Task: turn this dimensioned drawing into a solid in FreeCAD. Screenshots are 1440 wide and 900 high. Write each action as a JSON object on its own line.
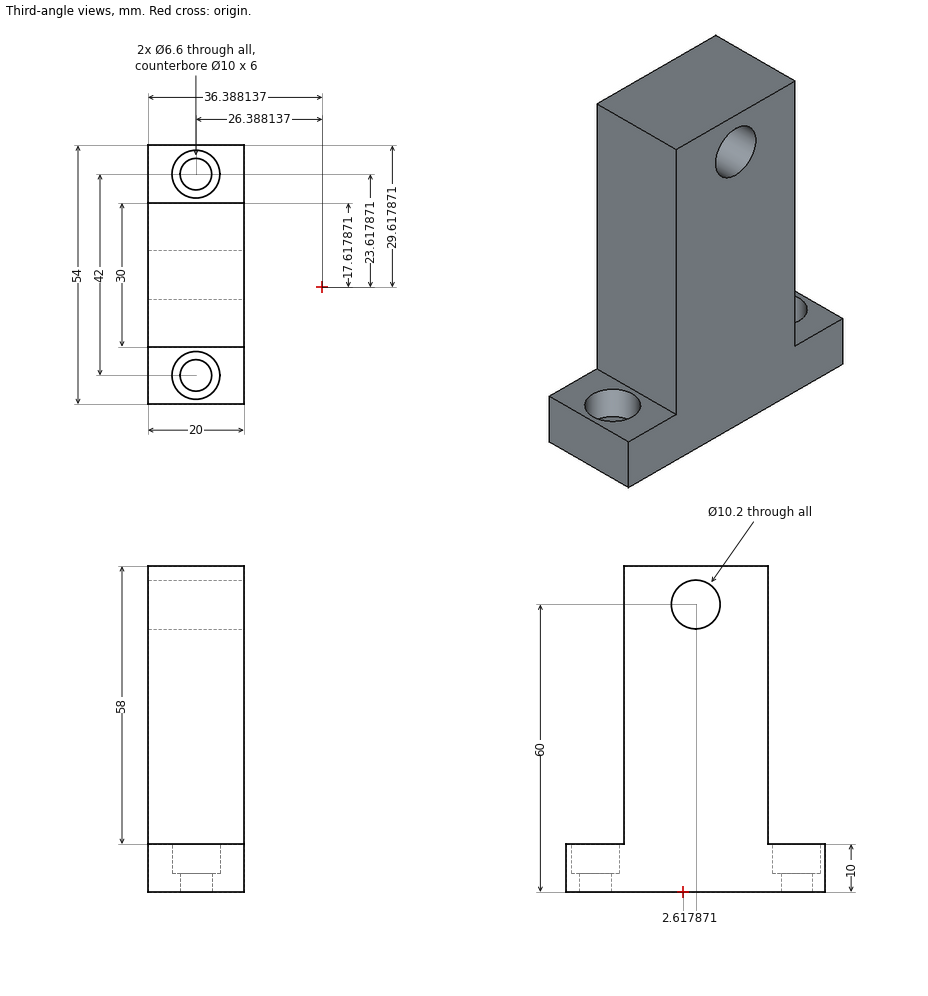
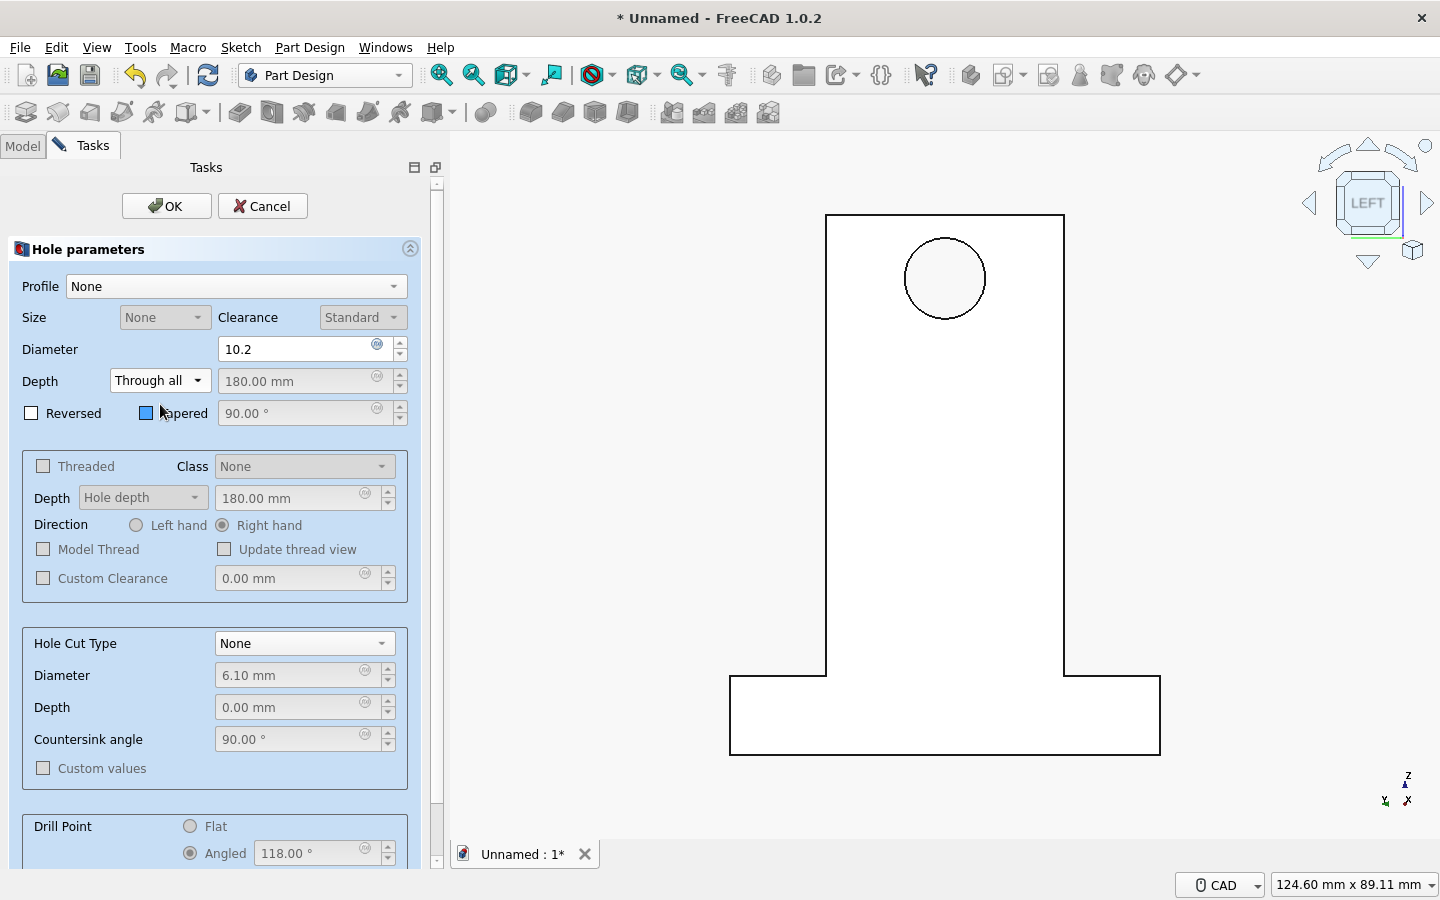
{"action": "left_click", "coordinate": [167, 206]}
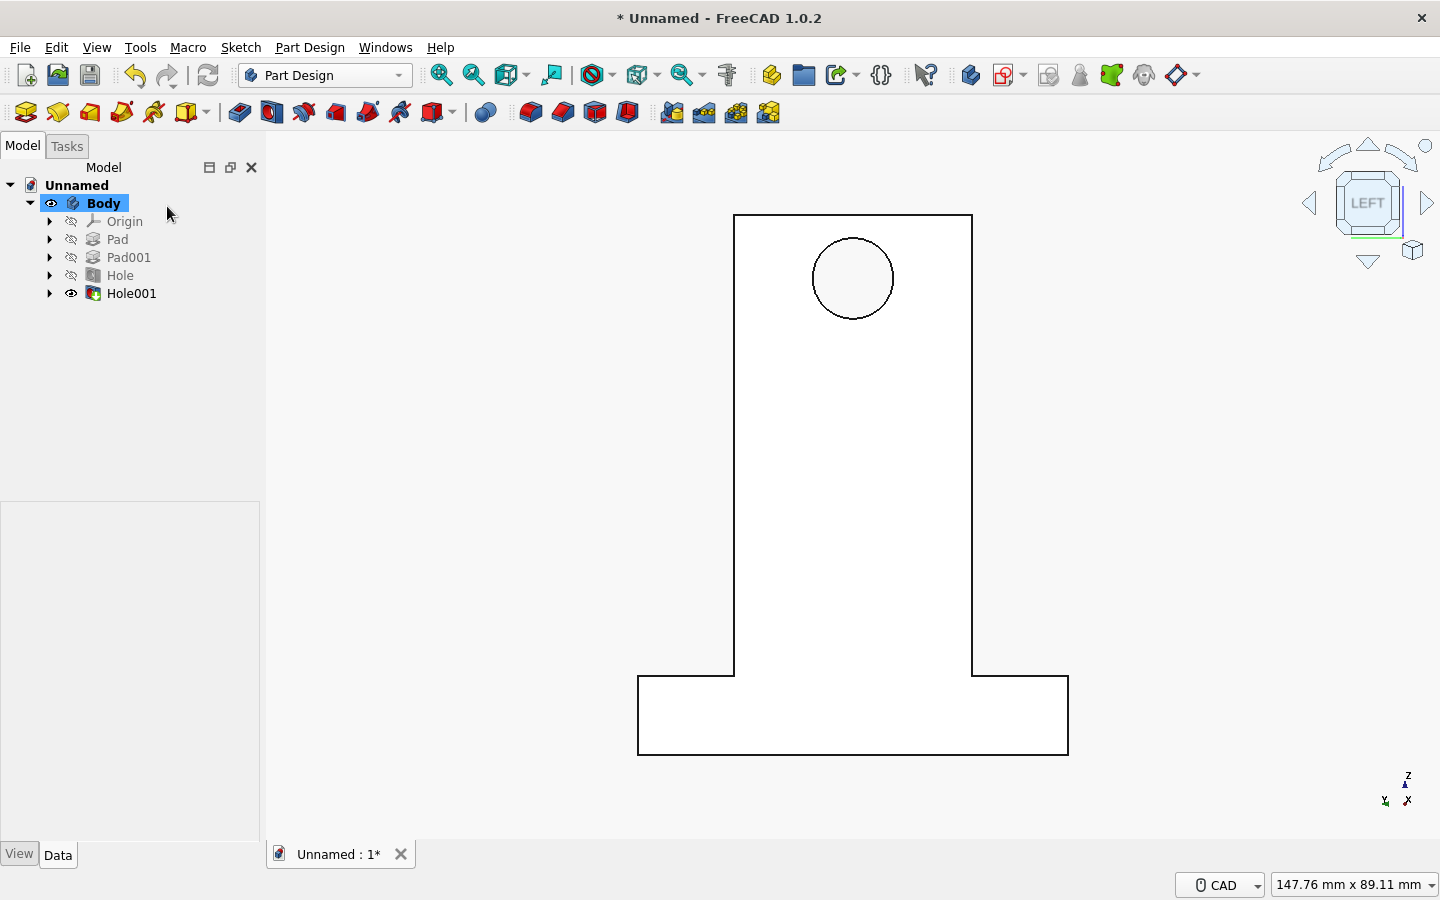
{"action": "key", "text": "0"}